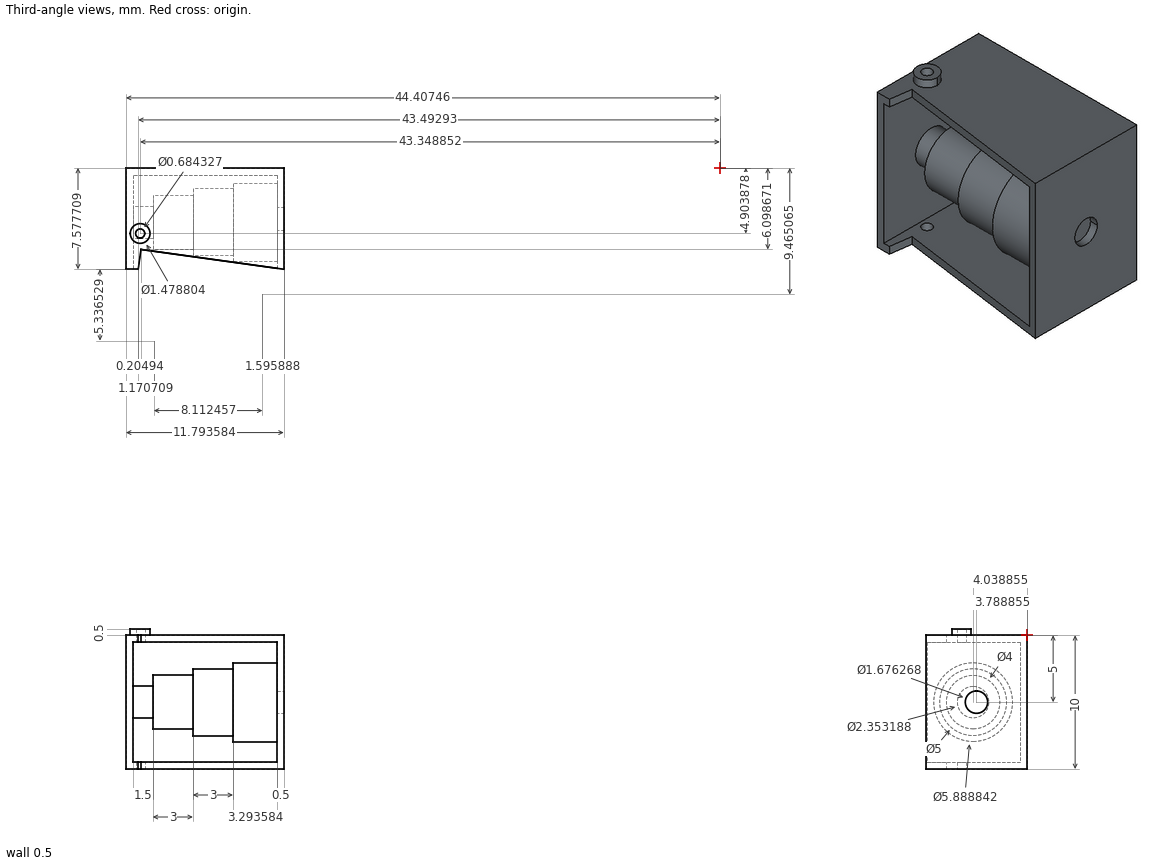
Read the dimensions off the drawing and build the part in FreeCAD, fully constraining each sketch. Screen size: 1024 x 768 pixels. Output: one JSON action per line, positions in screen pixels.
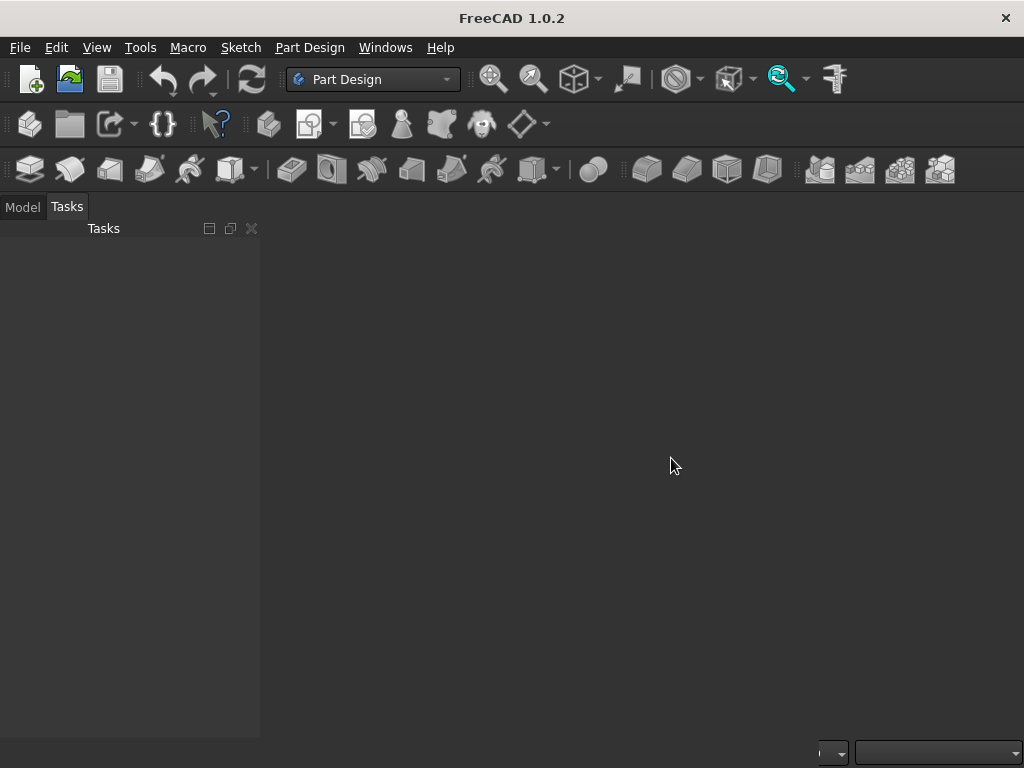
{"action": "left_click", "coordinate": [30, 80]}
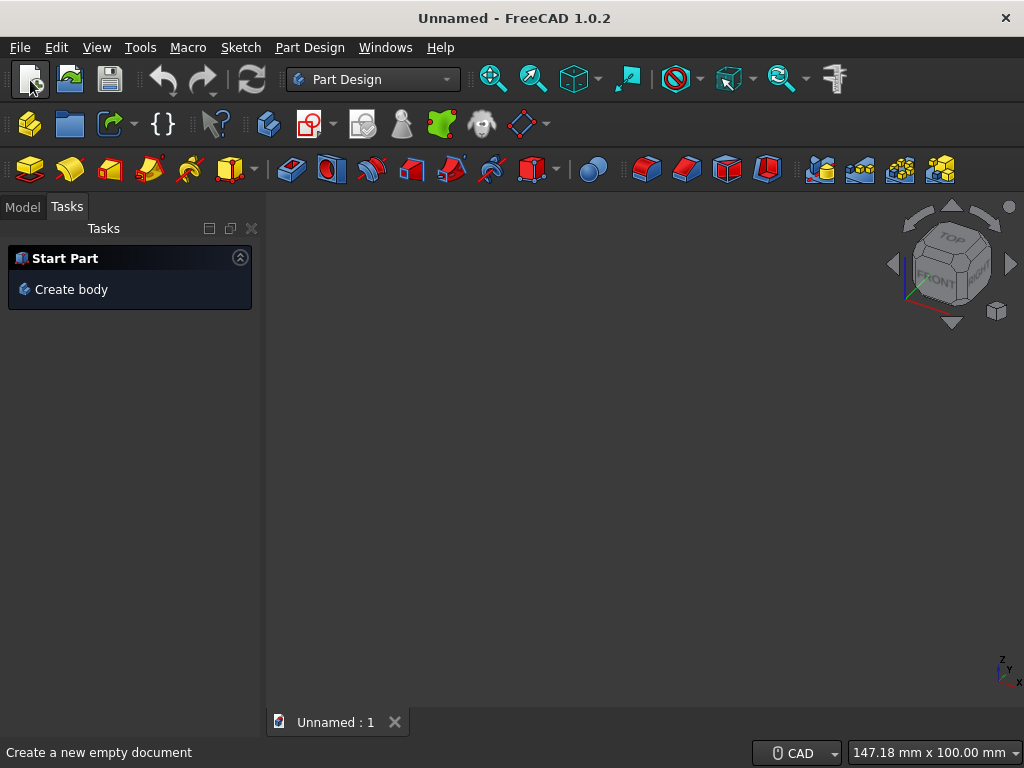
{"action": "left_click", "coordinate": [310, 124]}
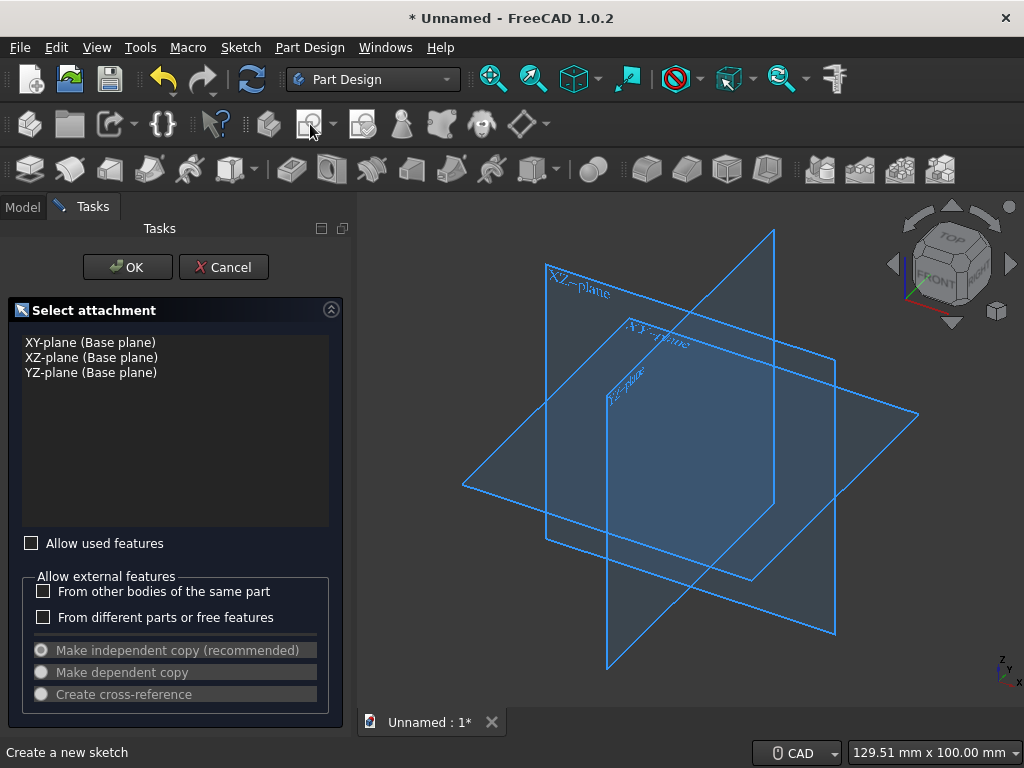
{"action": "left_click", "coordinate": [82, 342]}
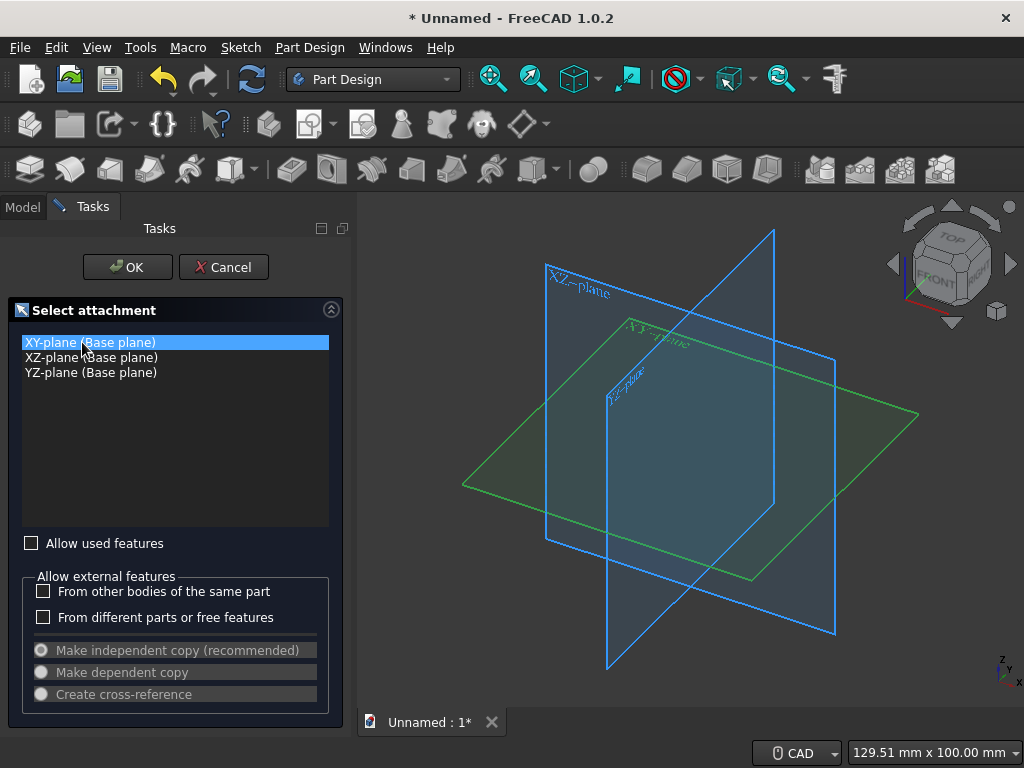
{"action": "left_click", "coordinate": [128, 267]}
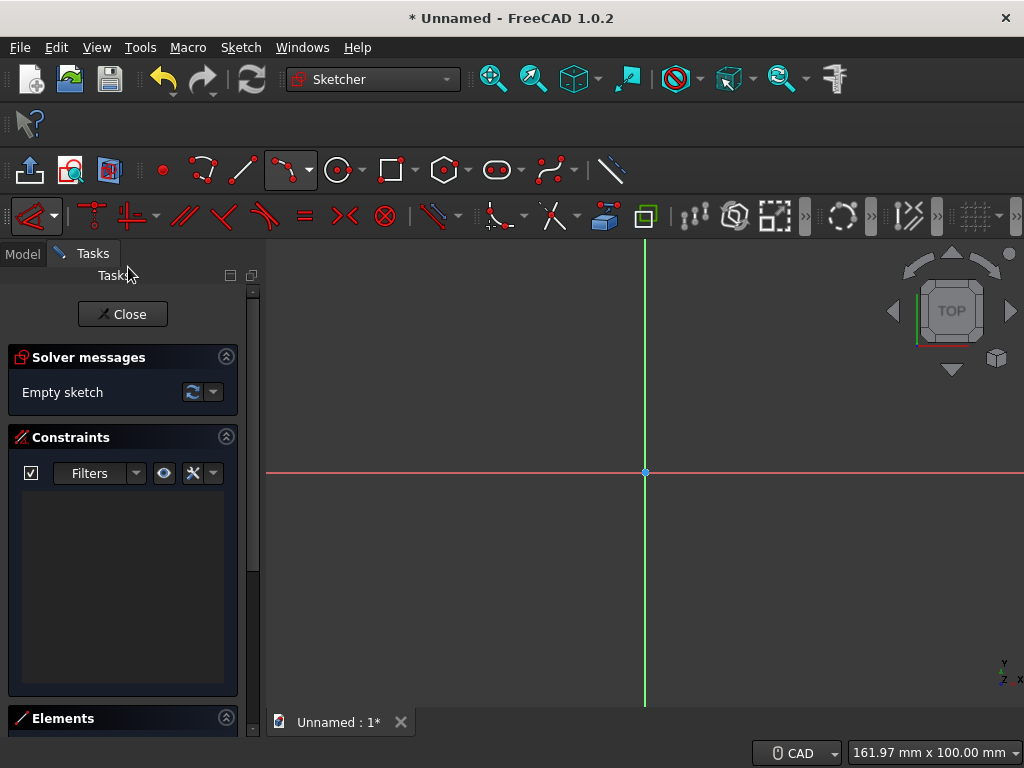
{"action": "scroll", "coordinate": [447, 494], "scroll_direction": "up", "scroll_amount": 10}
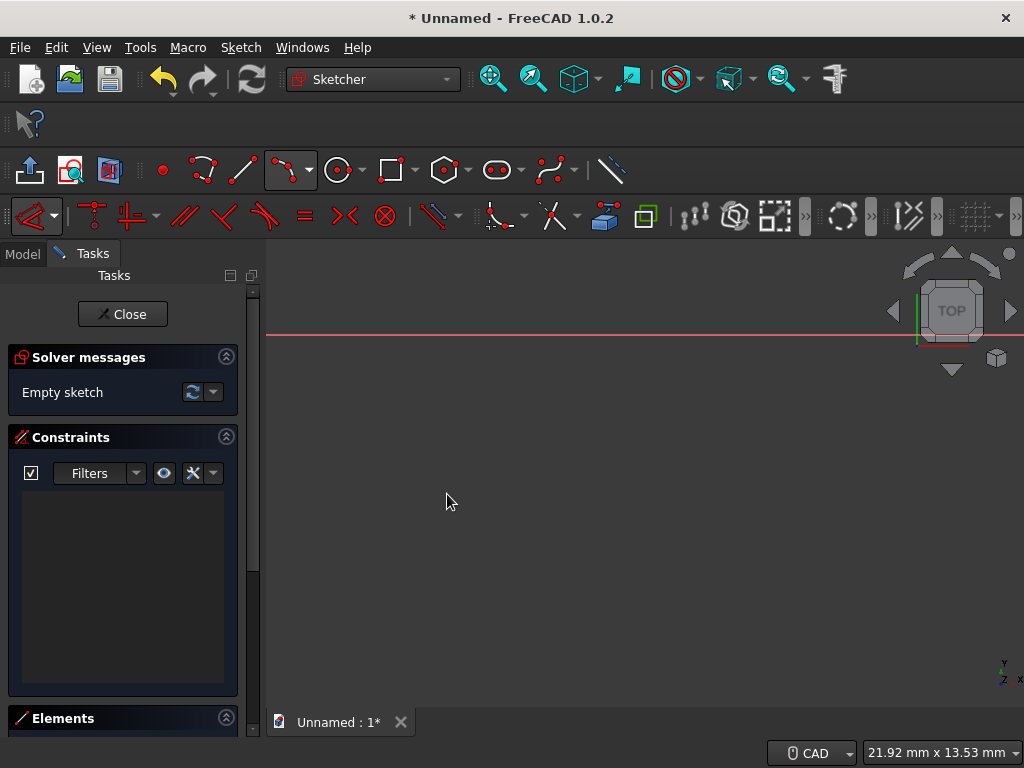
{"action": "left_click", "coordinate": [392, 170]}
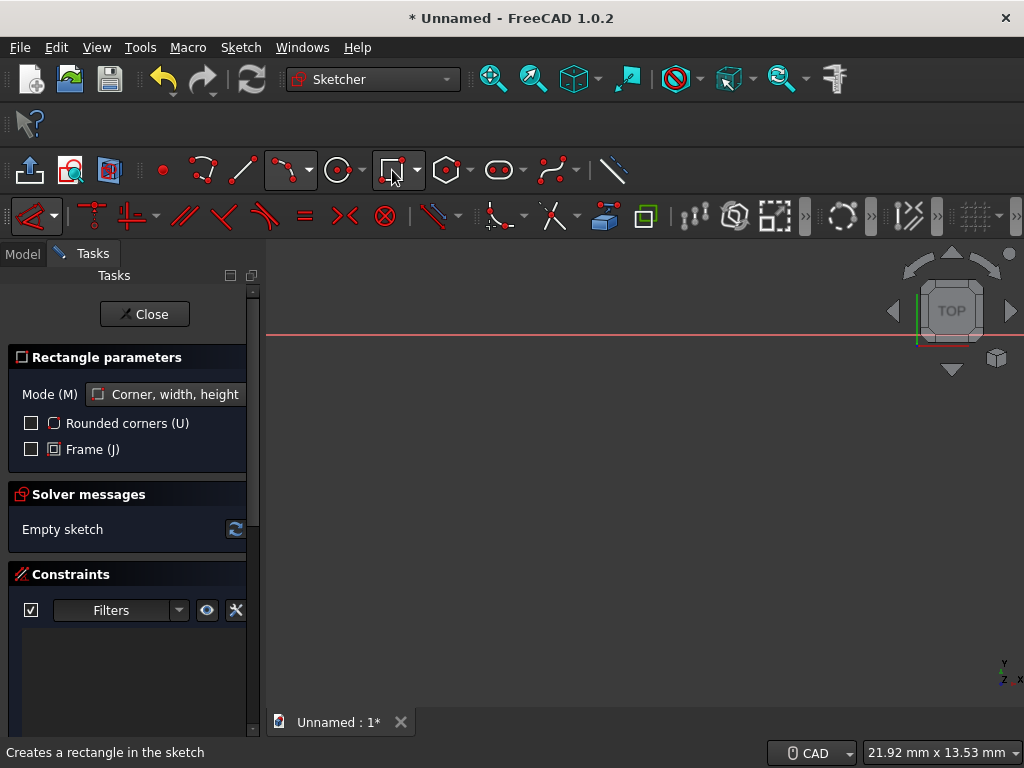
{"action": "left_click", "coordinate": [373, 335]}
{"action": "left_click", "coordinate": [781, 597]}
{"action": "key", "text": "Escape"}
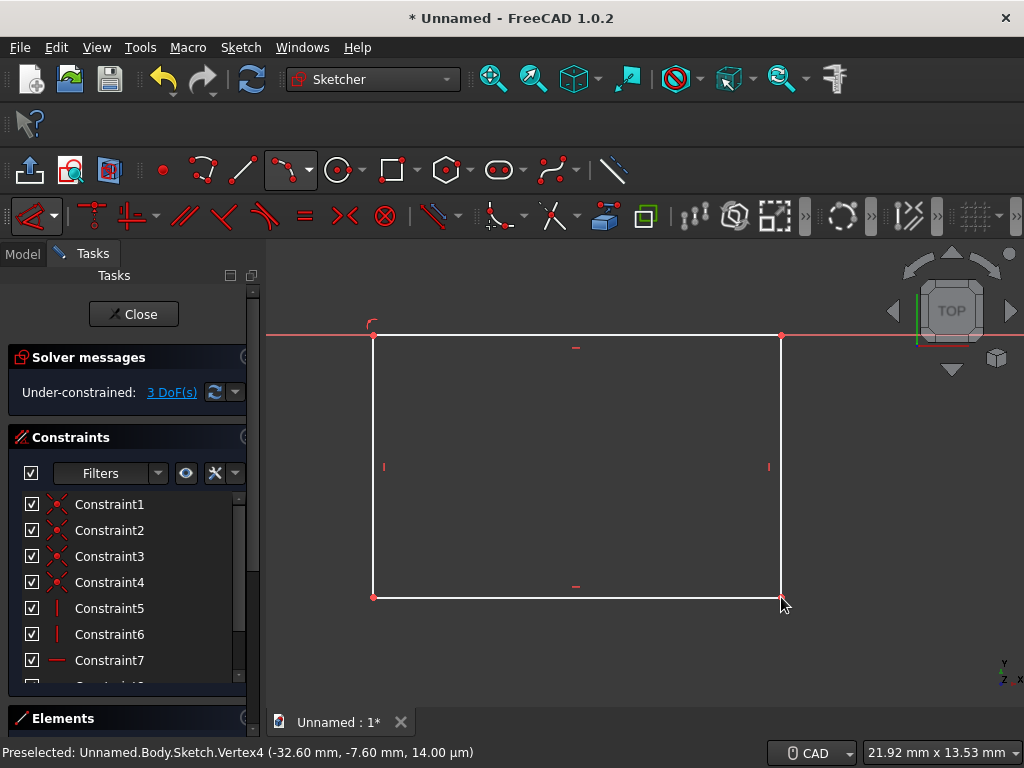
{"action": "left_click", "coordinate": [30, 216]}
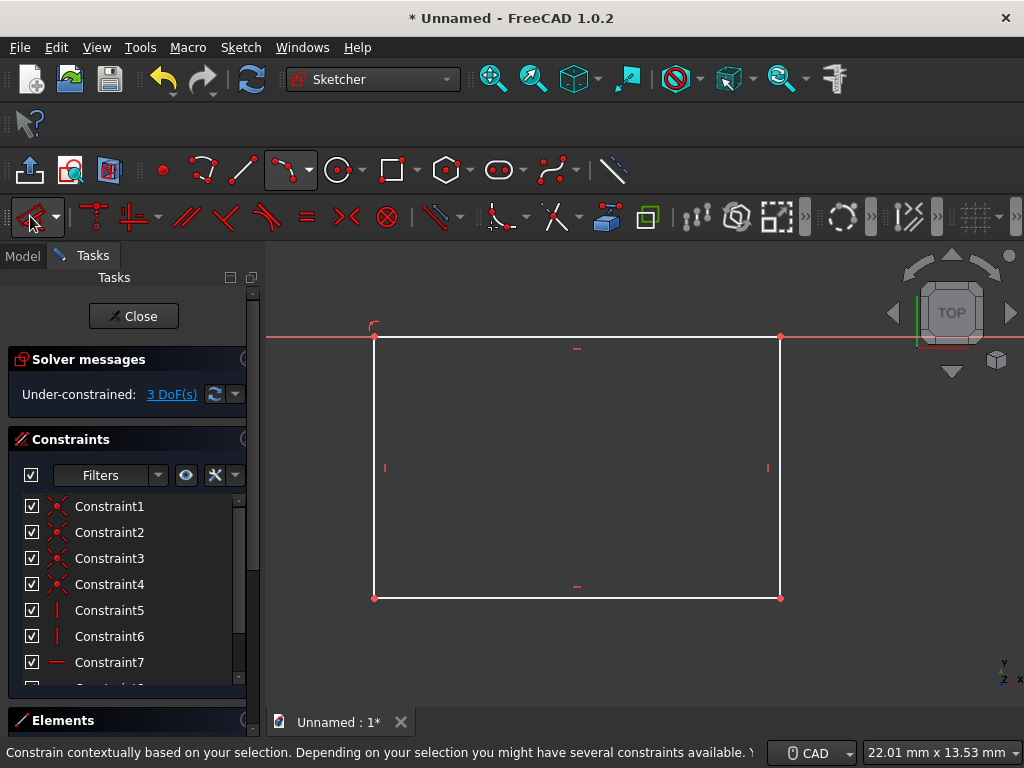
{"action": "left_click", "coordinate": [374, 415]}
{"action": "left_click", "coordinate": [340, 468]}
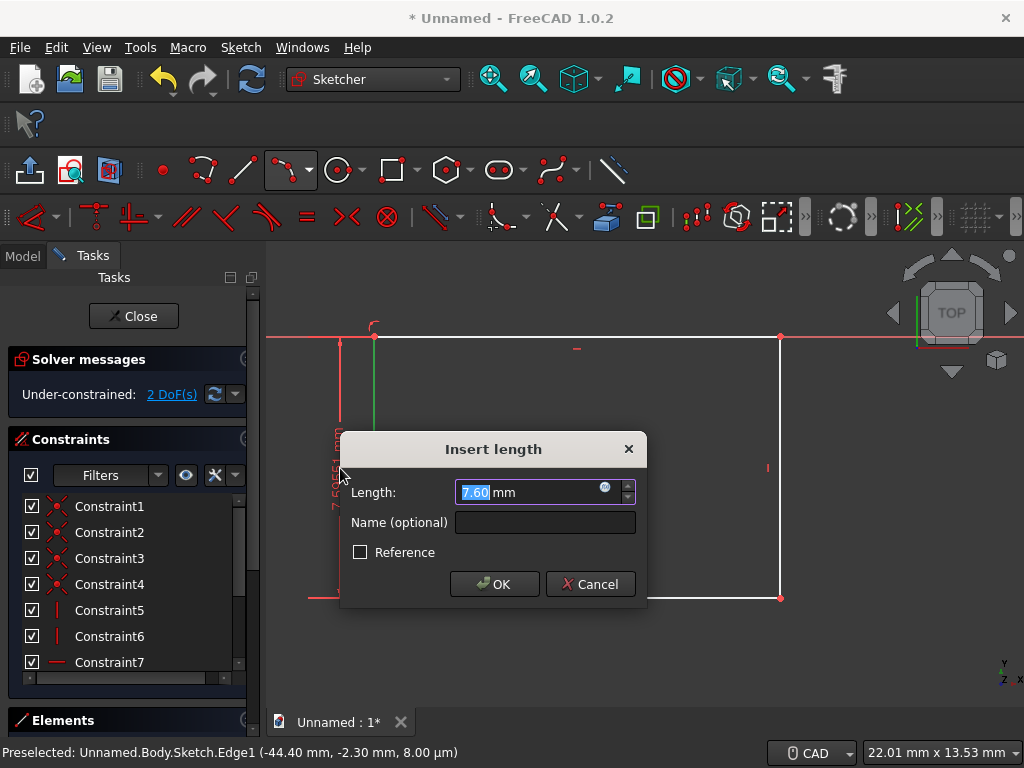
{"action": "type", "text": "7.577709"}
{"action": "key", "text": "Return"}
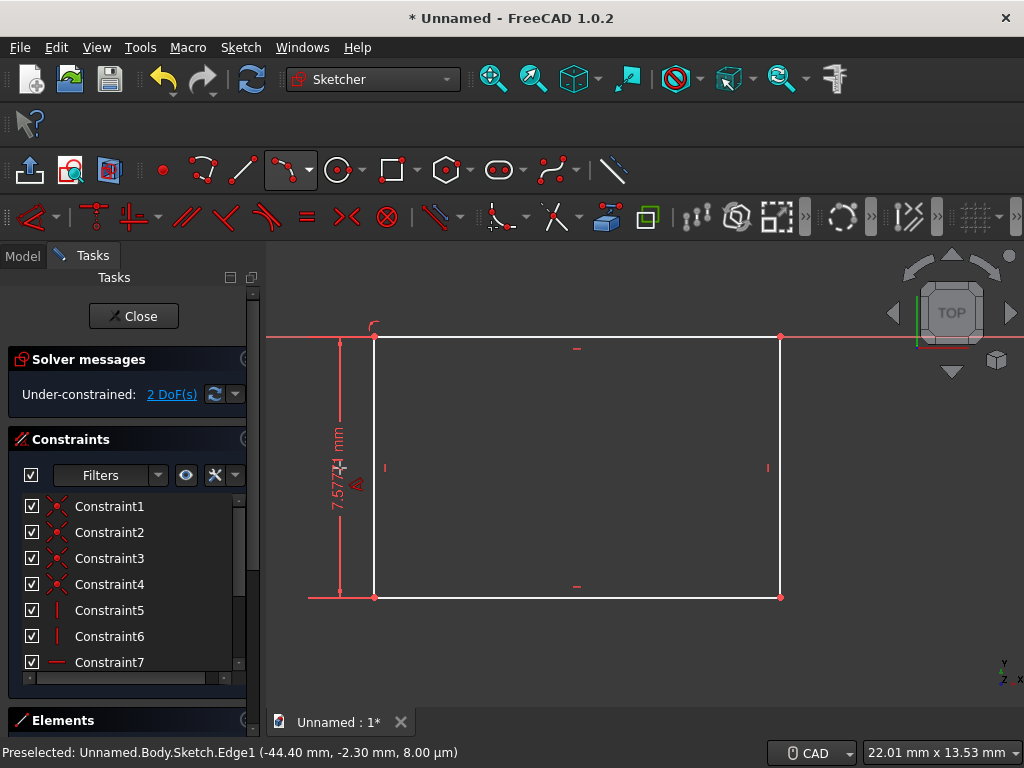
{"action": "left_click", "coordinate": [496, 598]}
{"action": "left_click", "coordinate": [577, 632]}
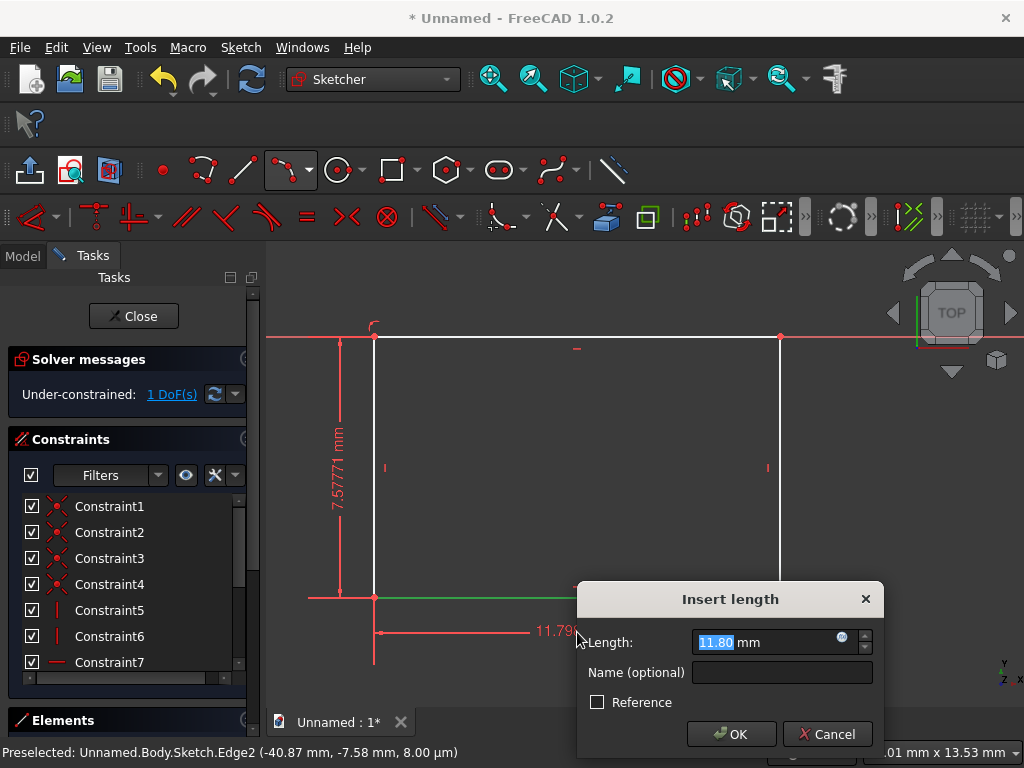
{"action": "type", "text": "11.793584"}
{"action": "key", "text": "Return"}